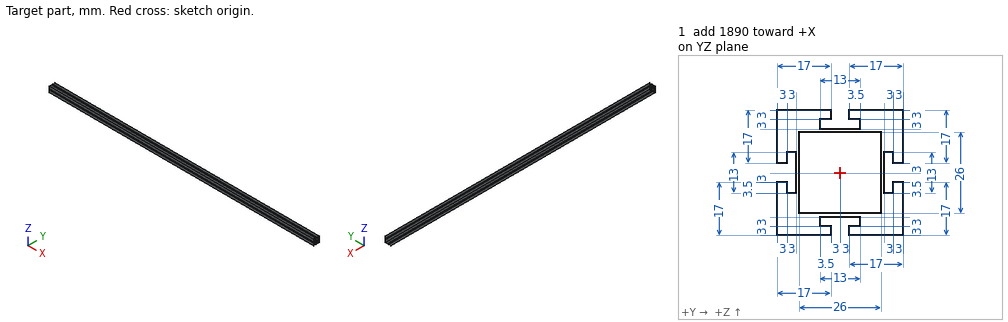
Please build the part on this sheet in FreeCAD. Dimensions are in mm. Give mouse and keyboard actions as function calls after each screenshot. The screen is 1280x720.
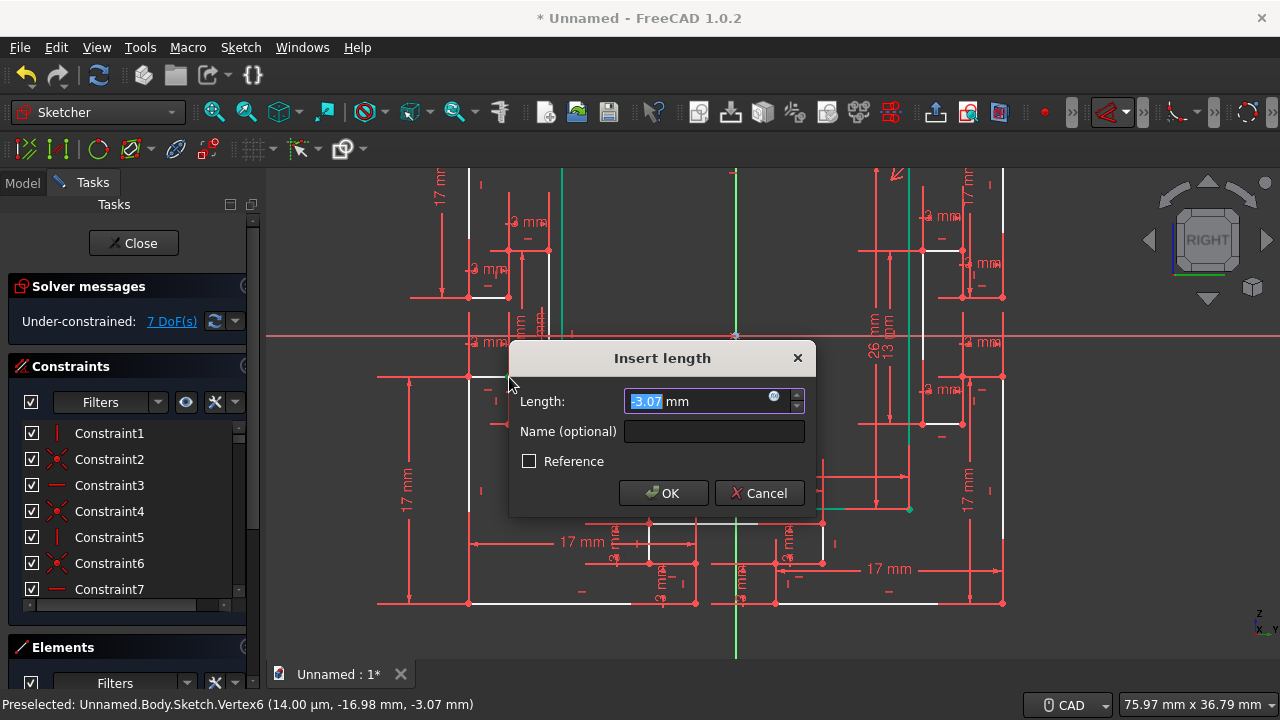
text(-3)
key(Return)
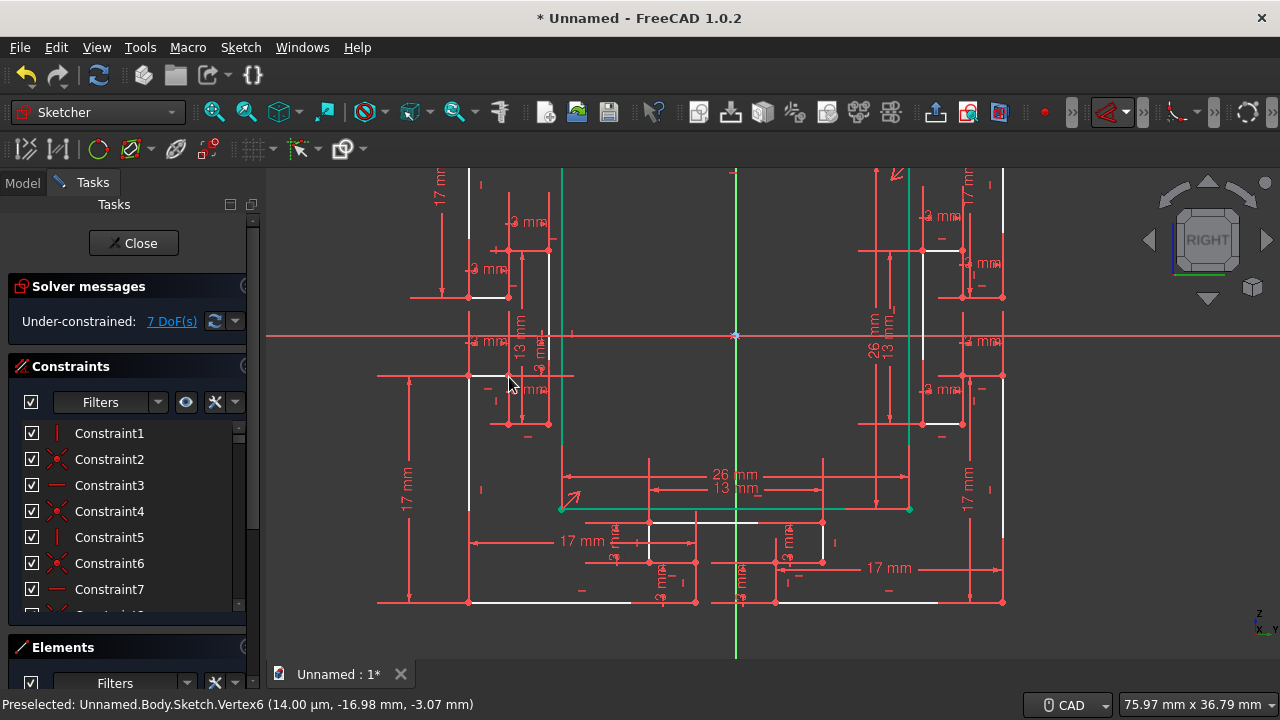
click(696, 603)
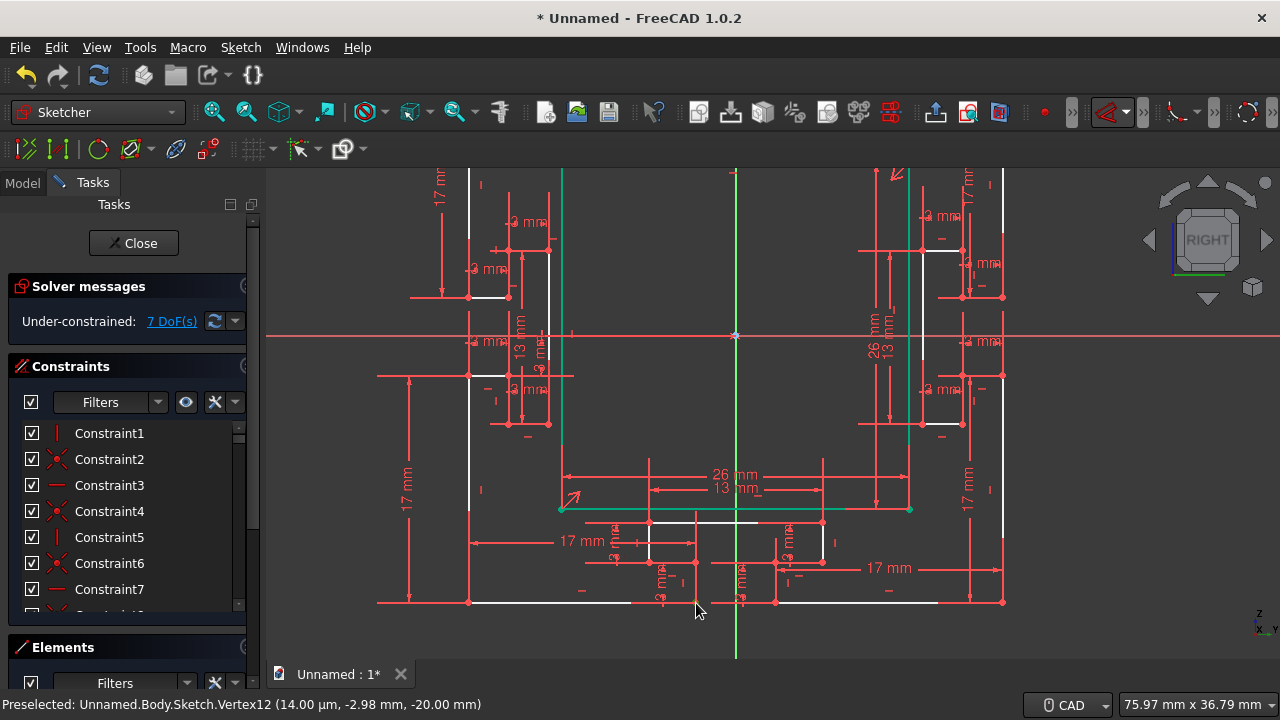
key(l)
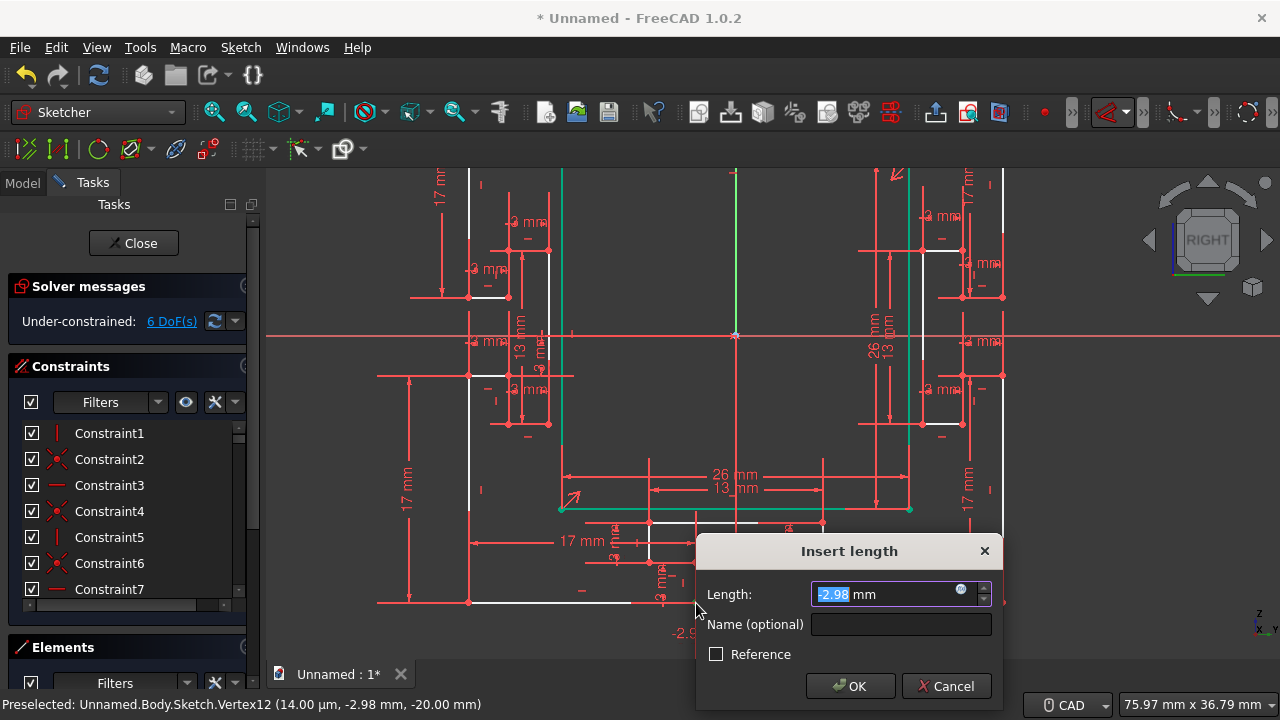
text(-3)
key(Return)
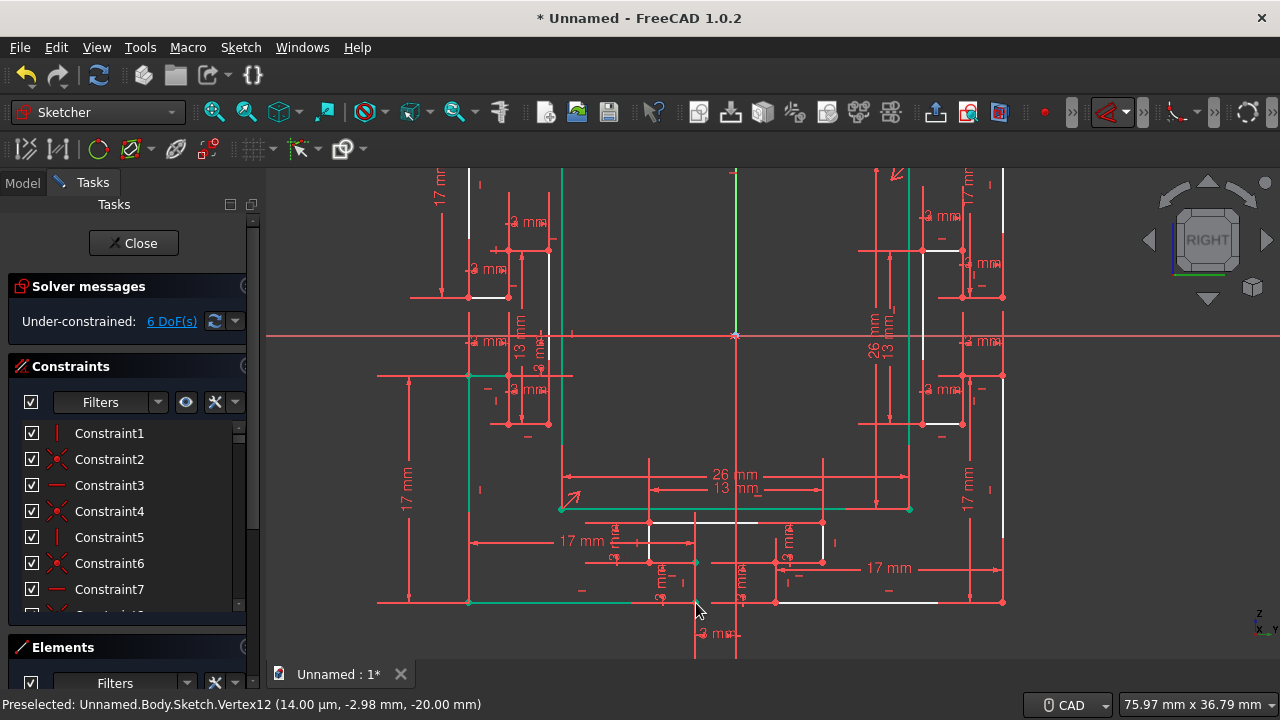
click(776, 563)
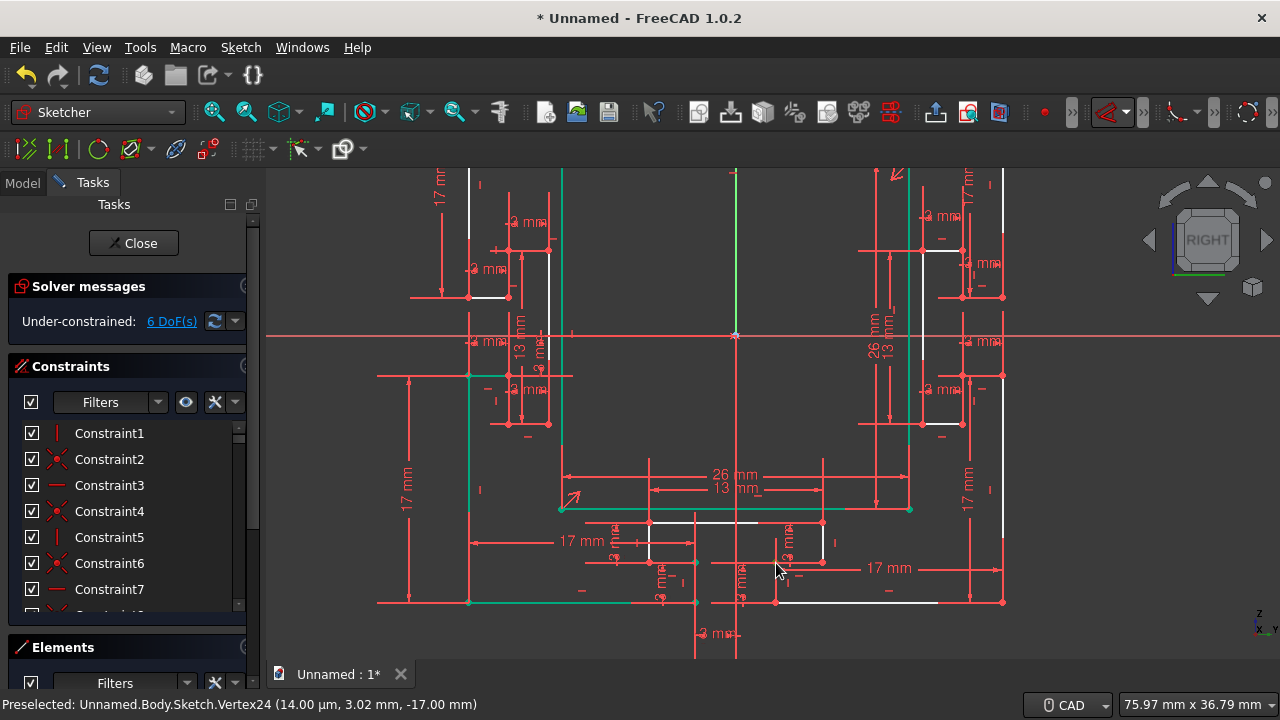
key(l)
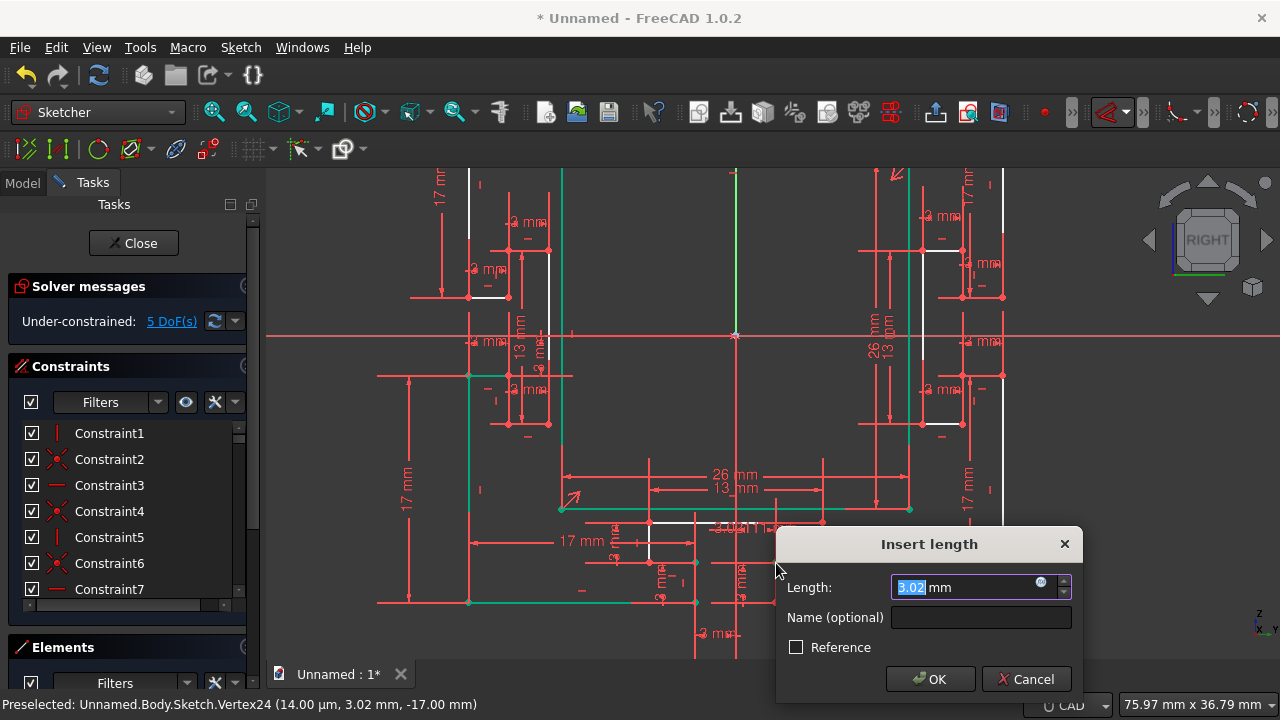
text(3)
key(Return)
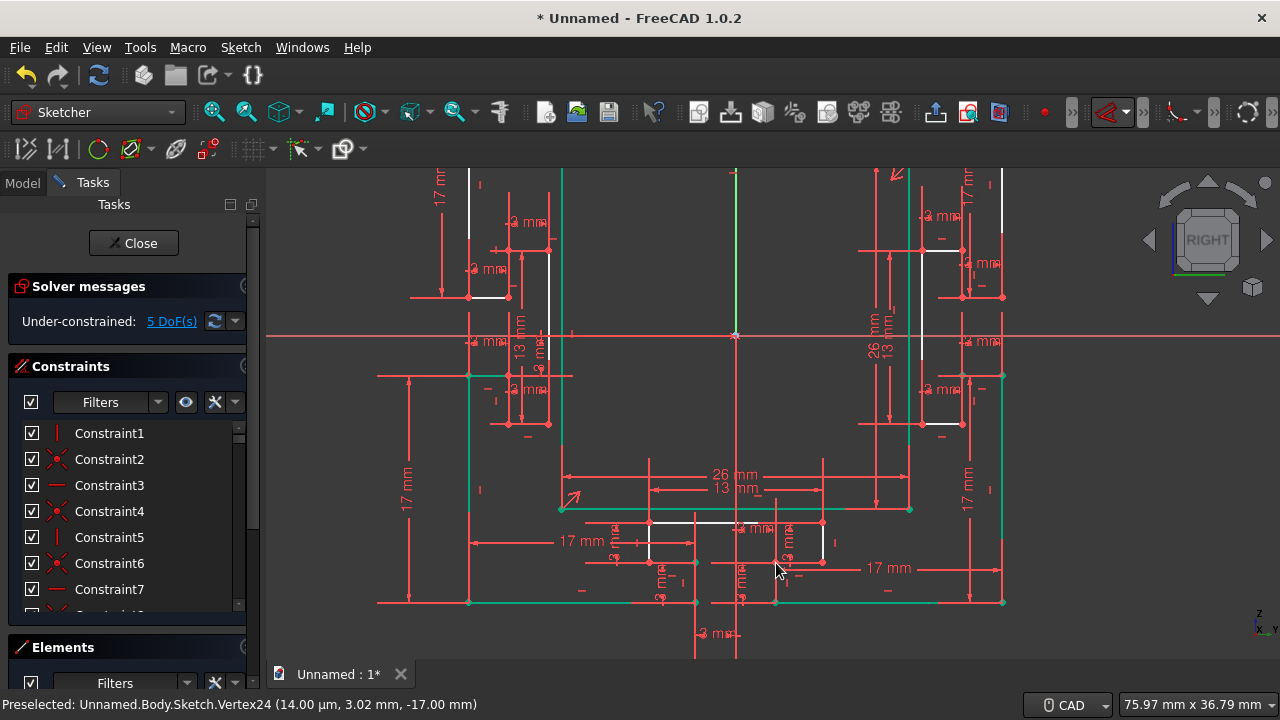
click(962, 298)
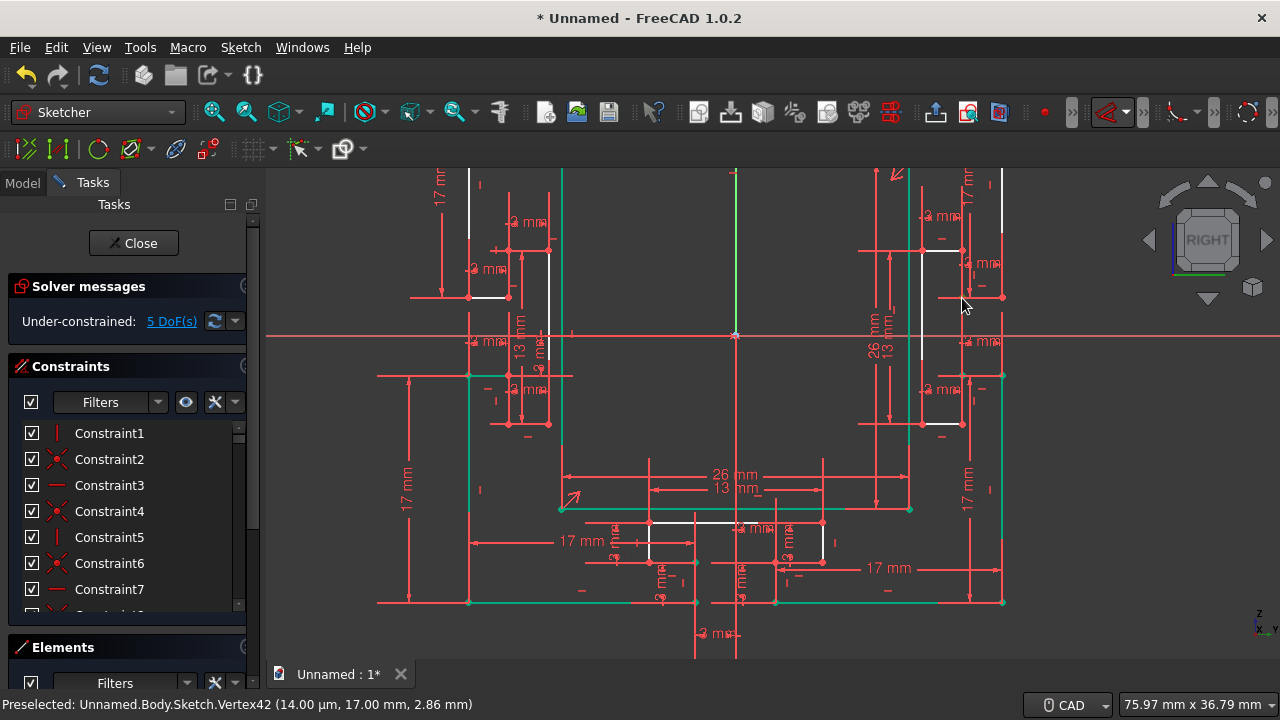
key(i)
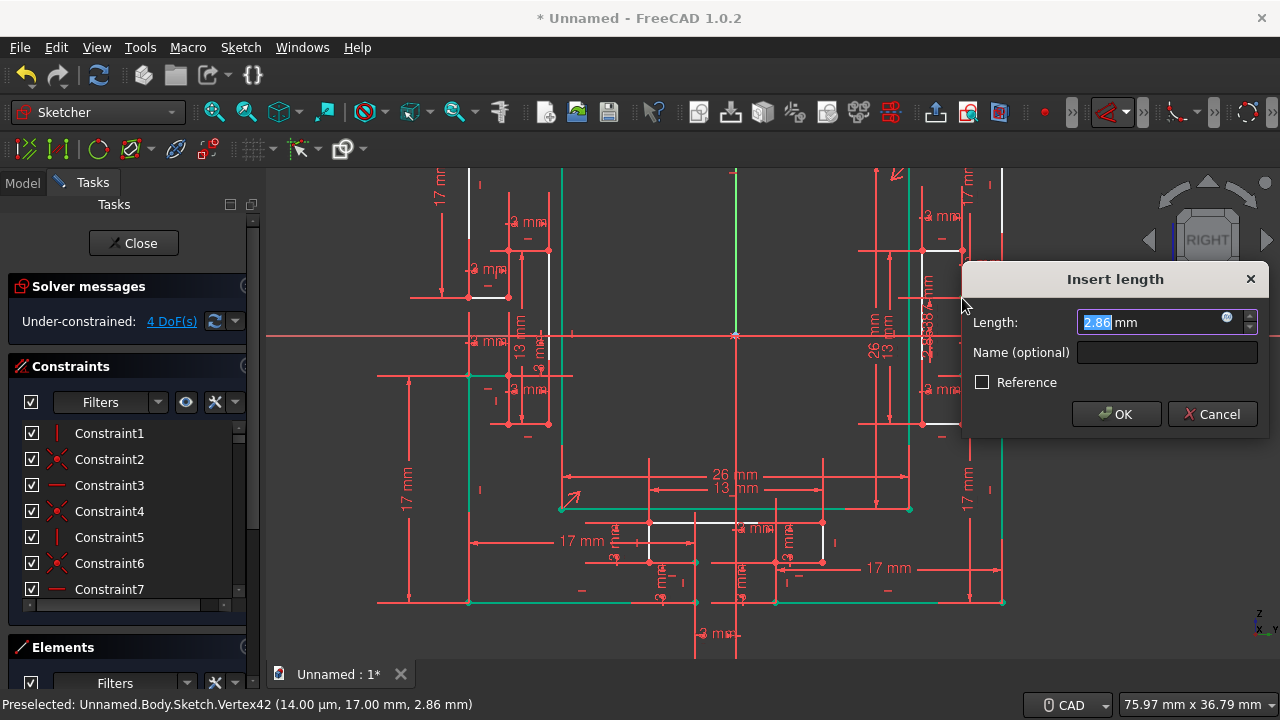
text(3)
key(Return)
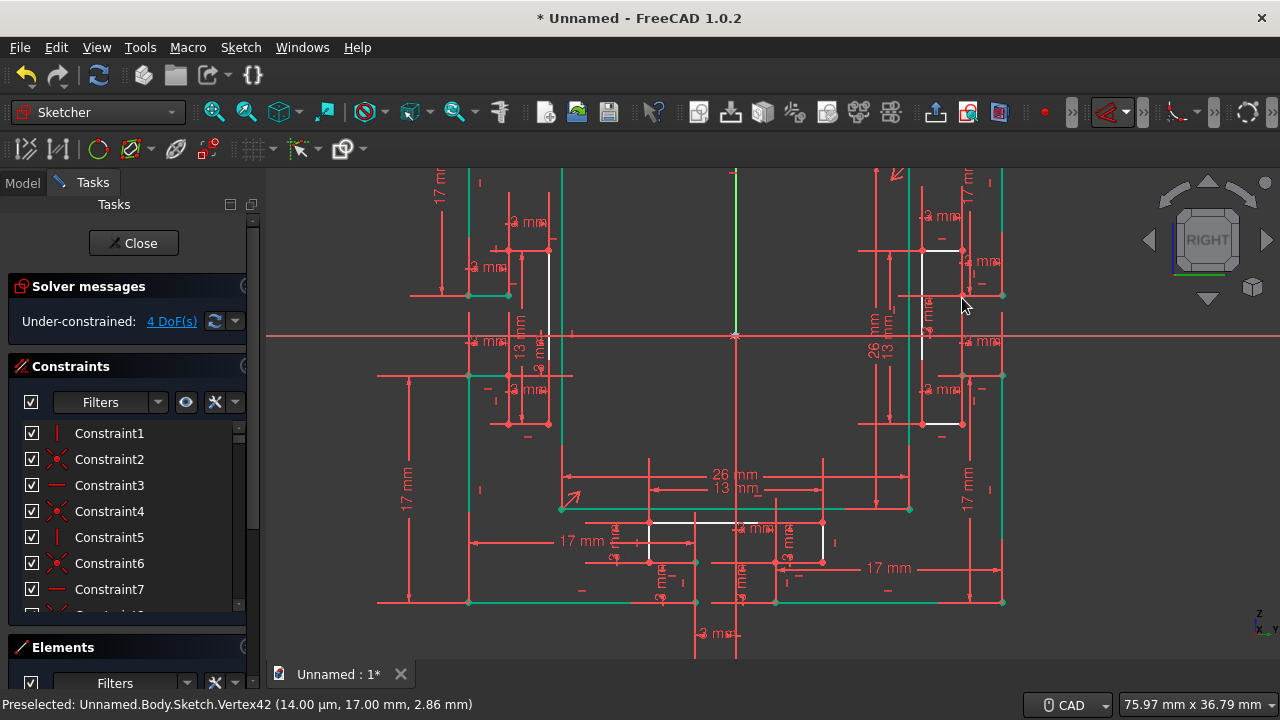
click(509, 410)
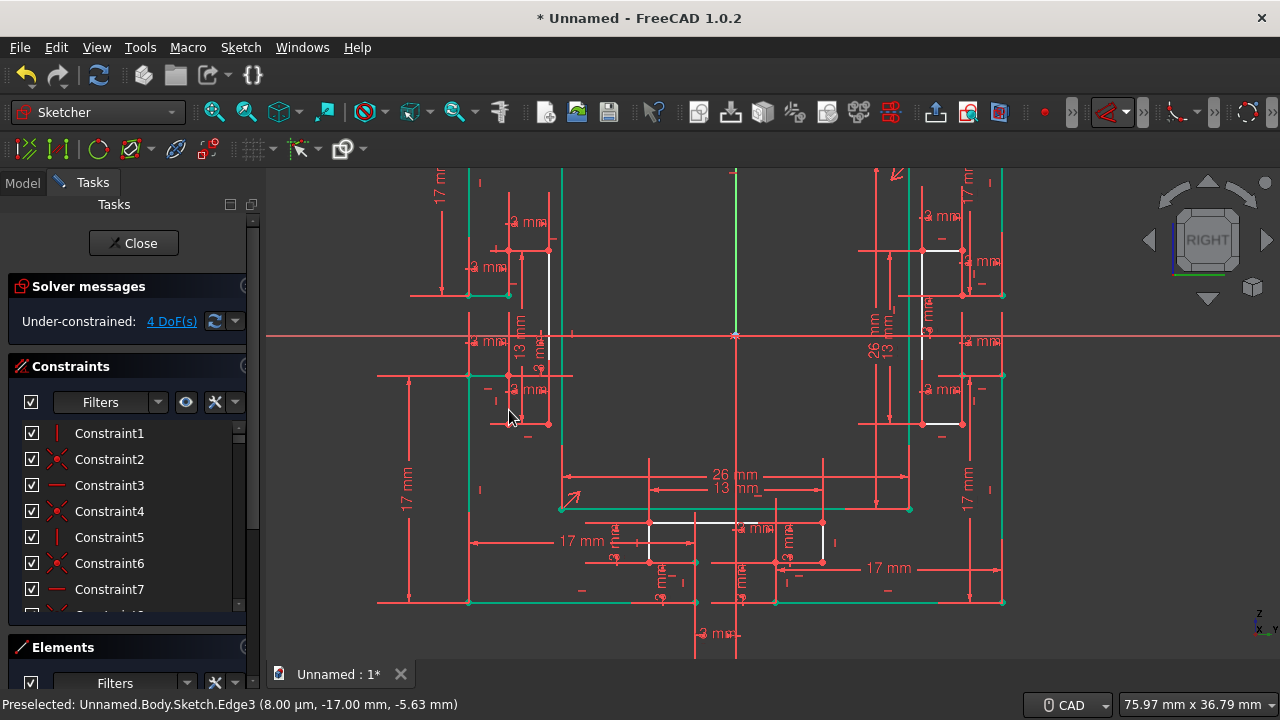
key(i)